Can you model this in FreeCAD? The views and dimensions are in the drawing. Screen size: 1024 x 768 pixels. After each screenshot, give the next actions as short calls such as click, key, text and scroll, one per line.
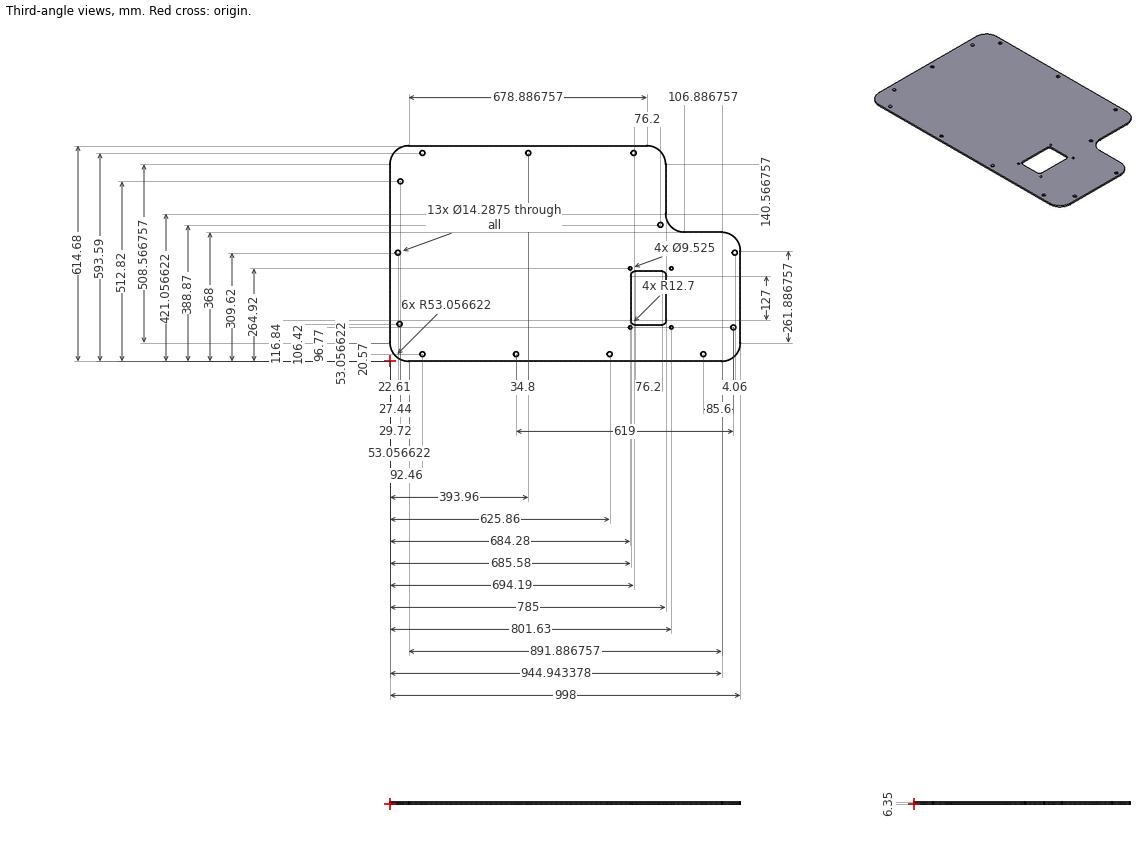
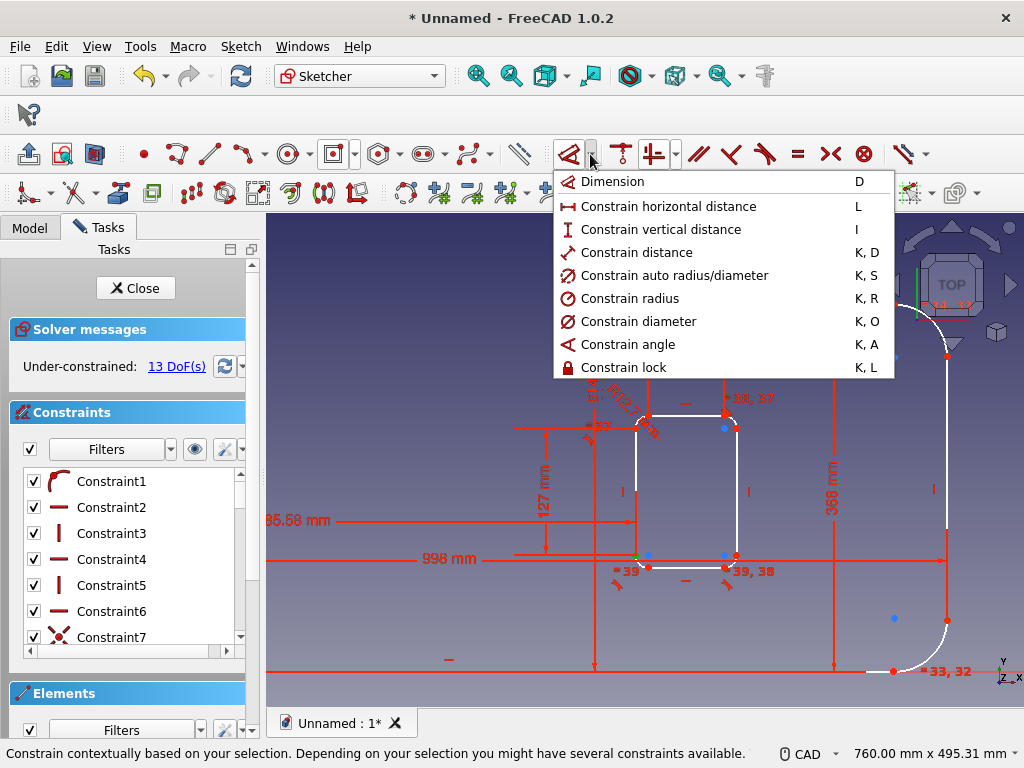
click(724, 230)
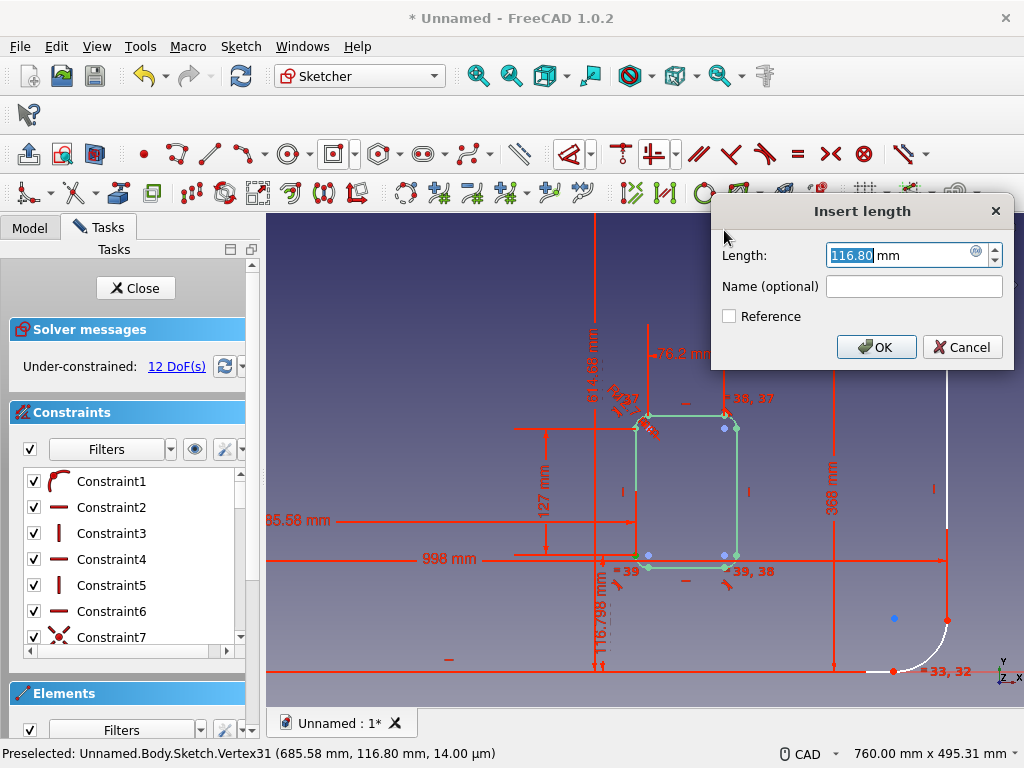
text(116.84)
key(Return)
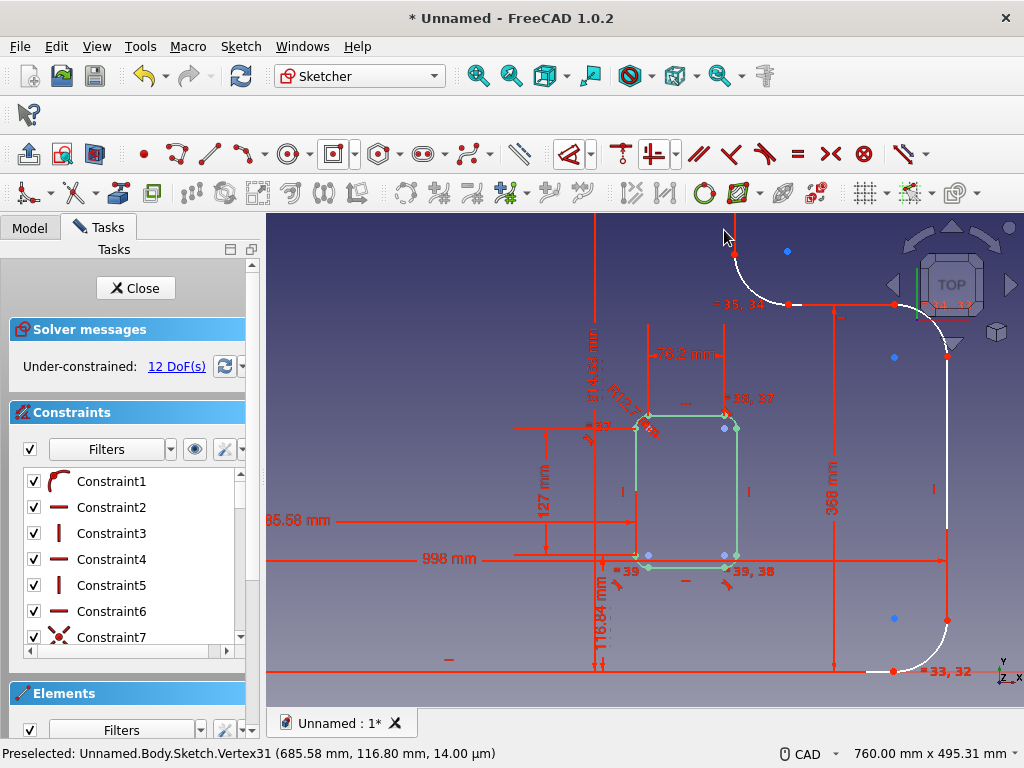
scroll(650, 515, down, 5)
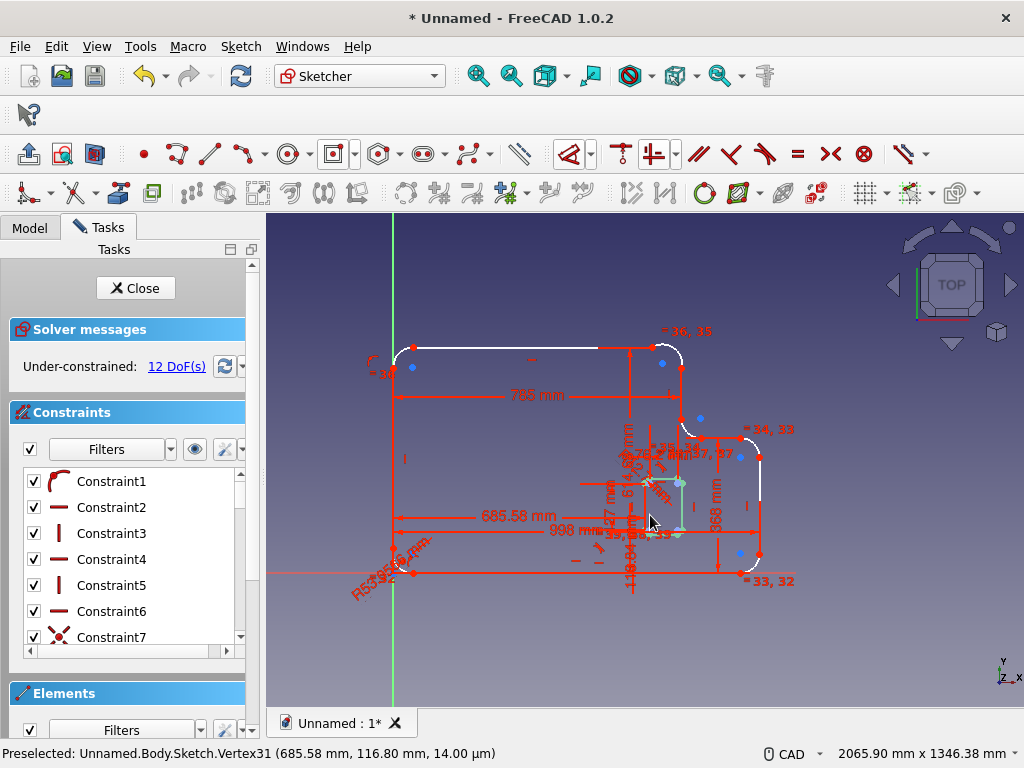
click(393, 422)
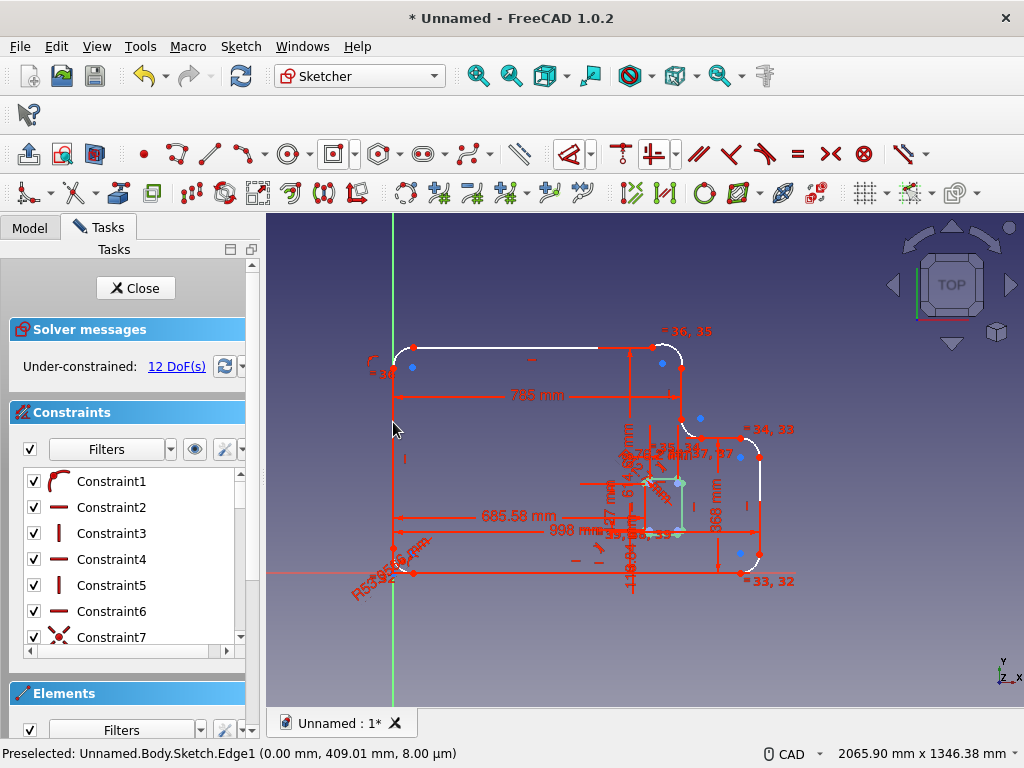
click(590, 154)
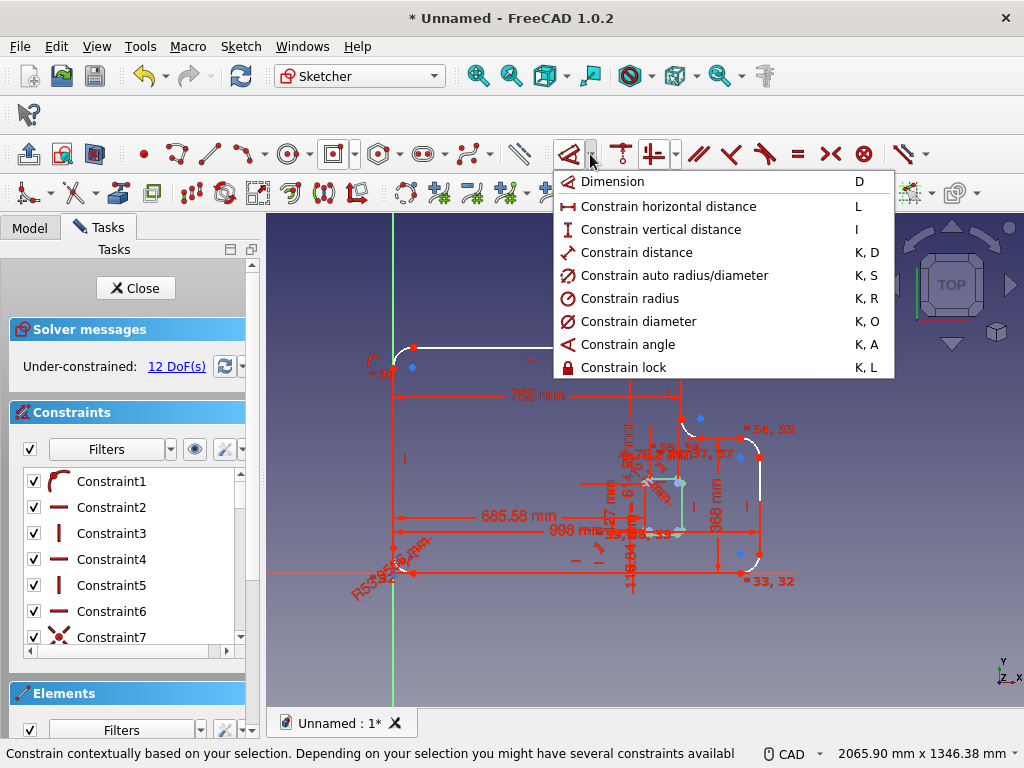
click(724, 230)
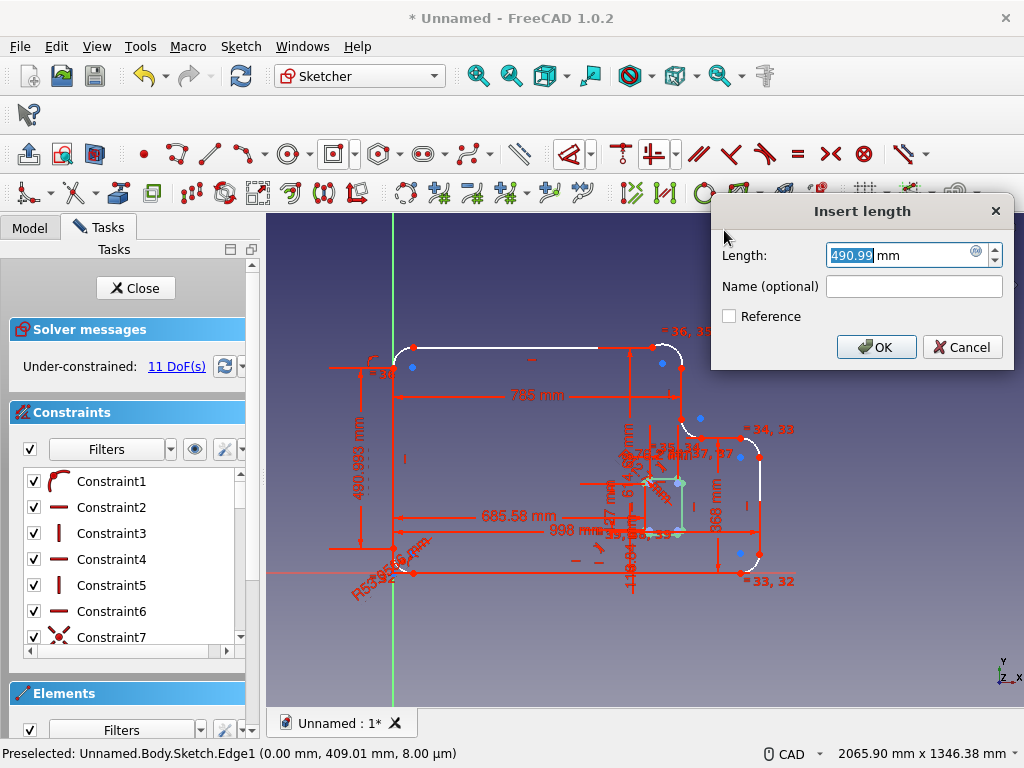
text(508.566757)
key(Return)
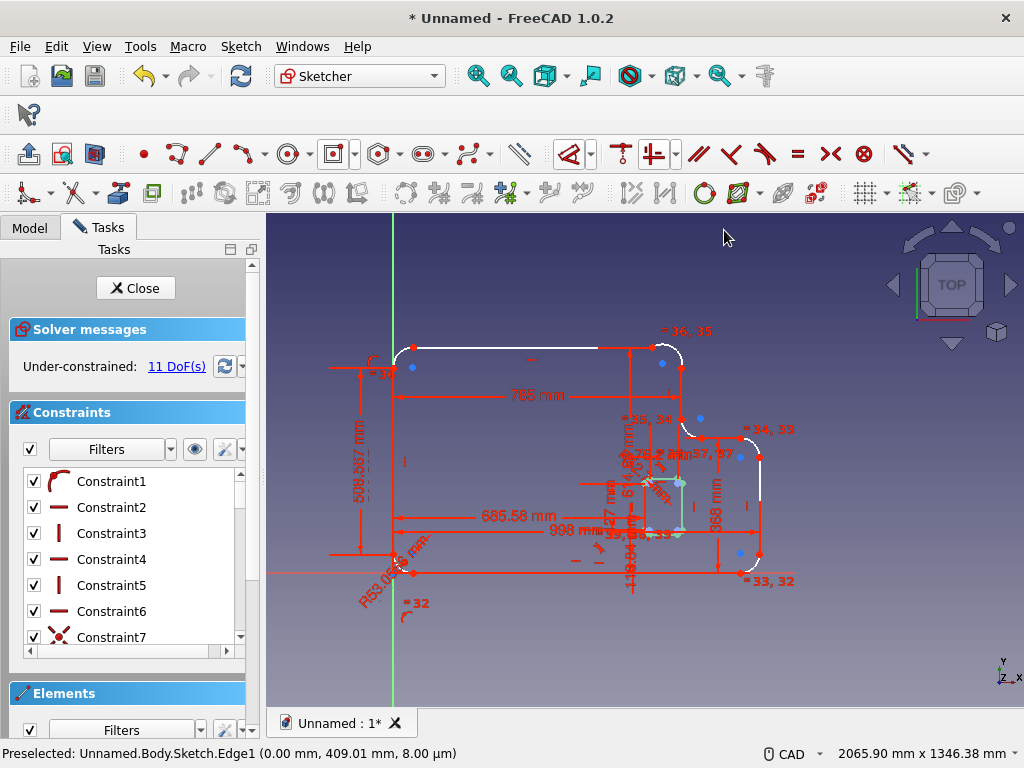
click(511, 573)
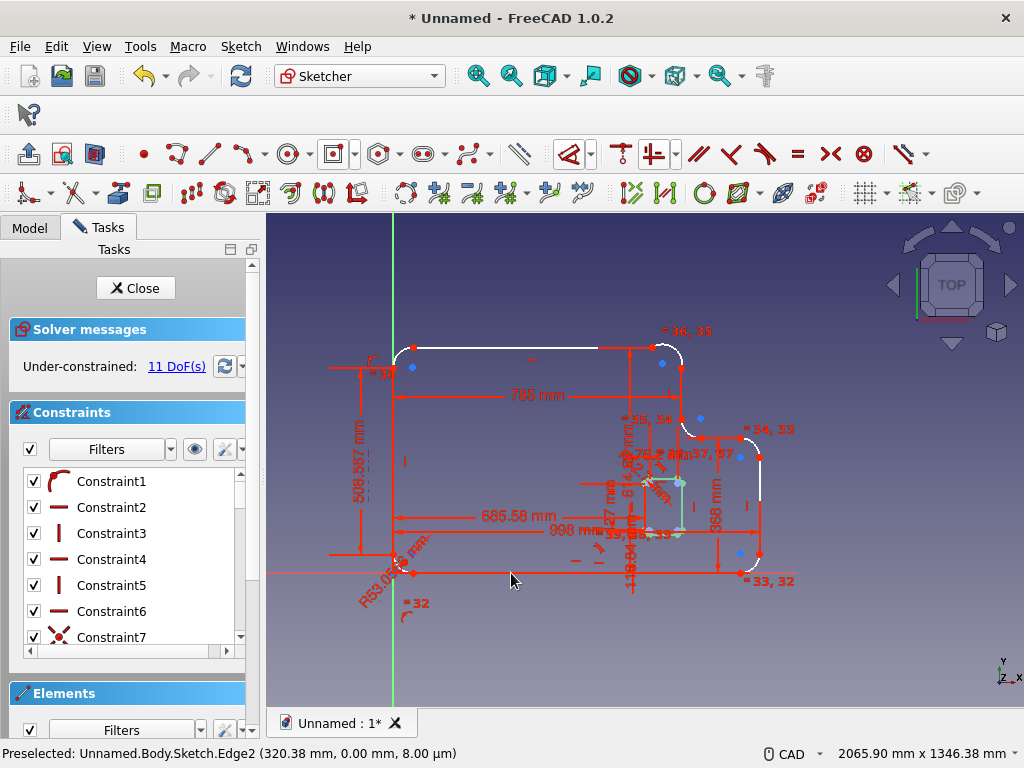
click(590, 154)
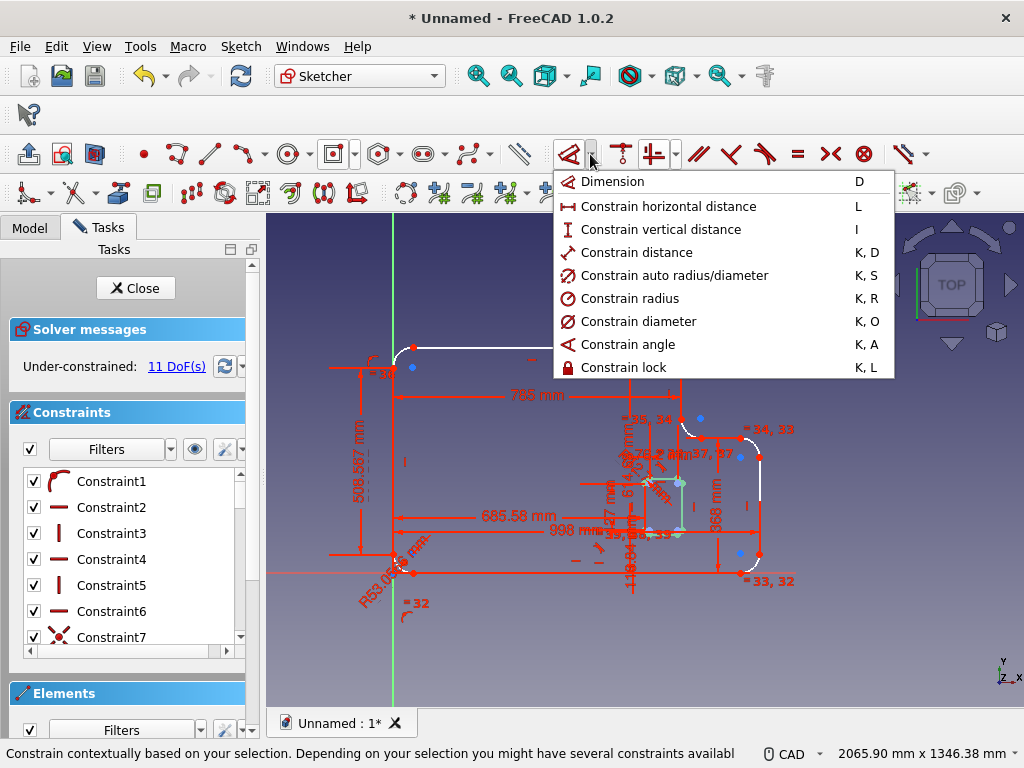
click(724, 206)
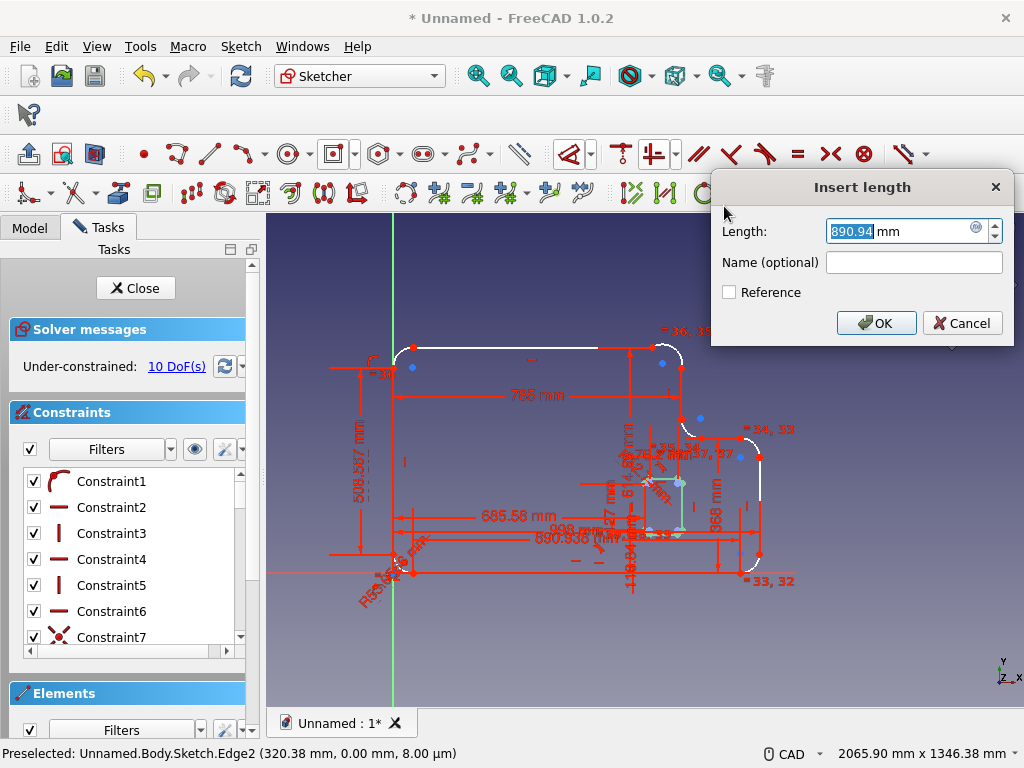
text(891.886757)
key(Return)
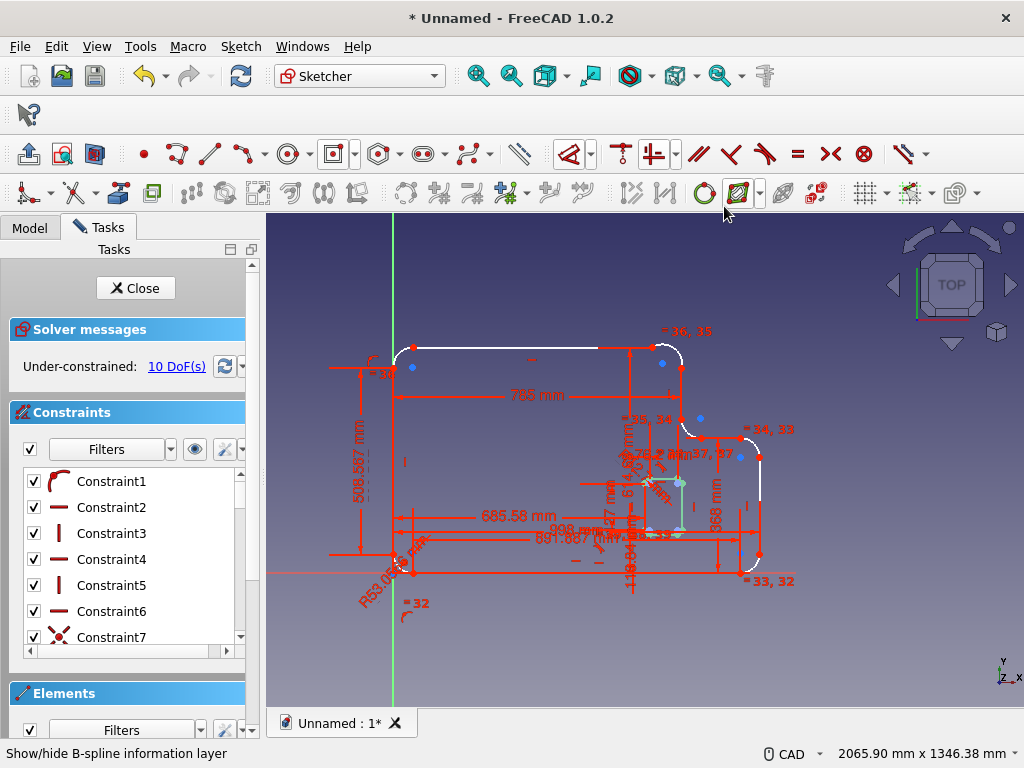
click(760, 525)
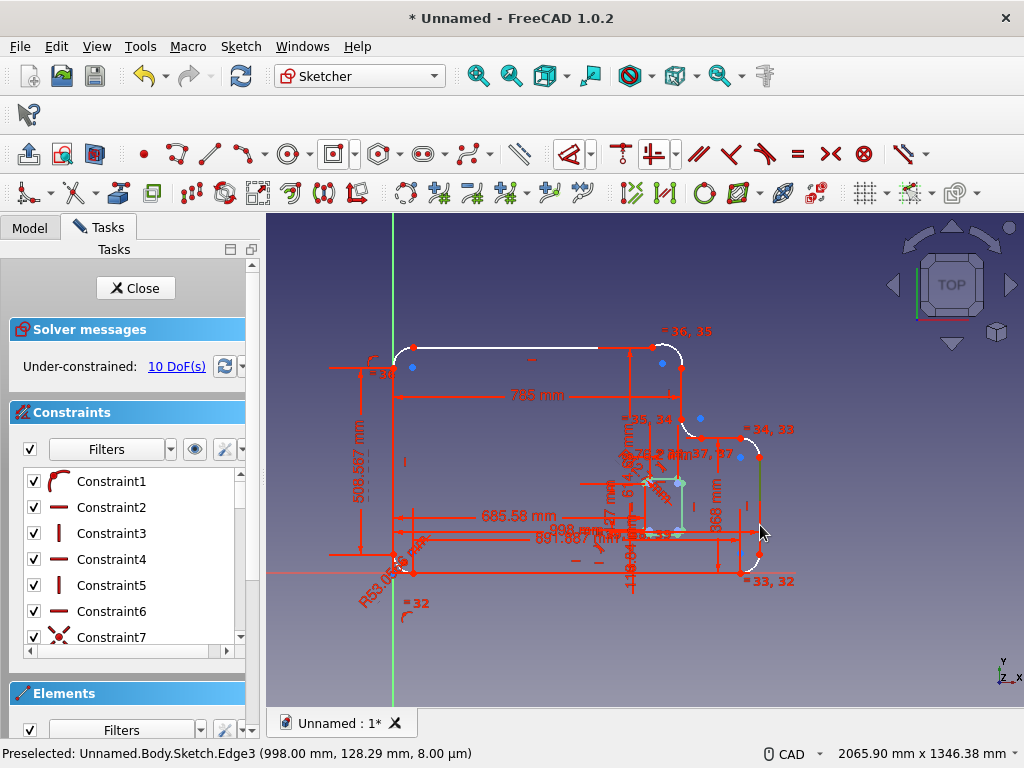
key(i)